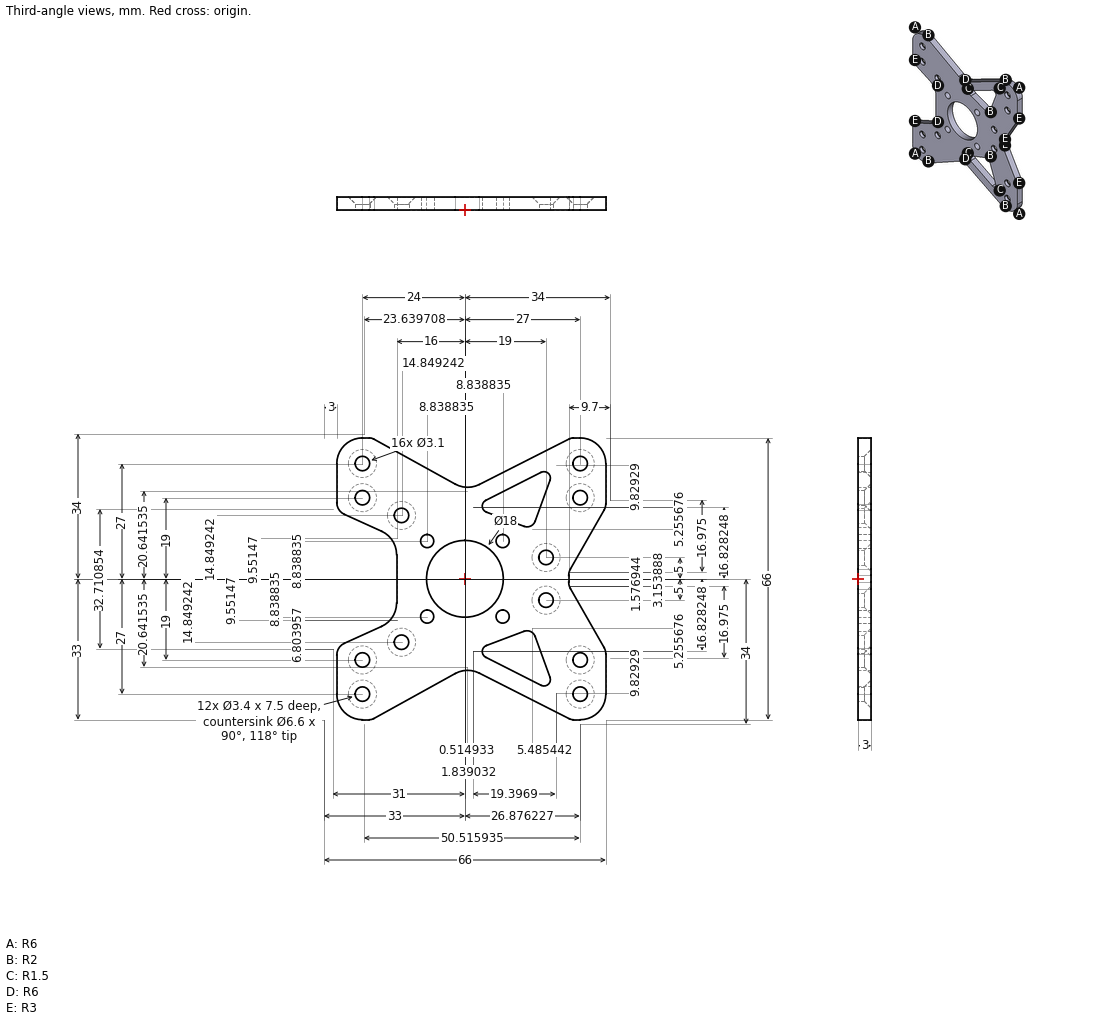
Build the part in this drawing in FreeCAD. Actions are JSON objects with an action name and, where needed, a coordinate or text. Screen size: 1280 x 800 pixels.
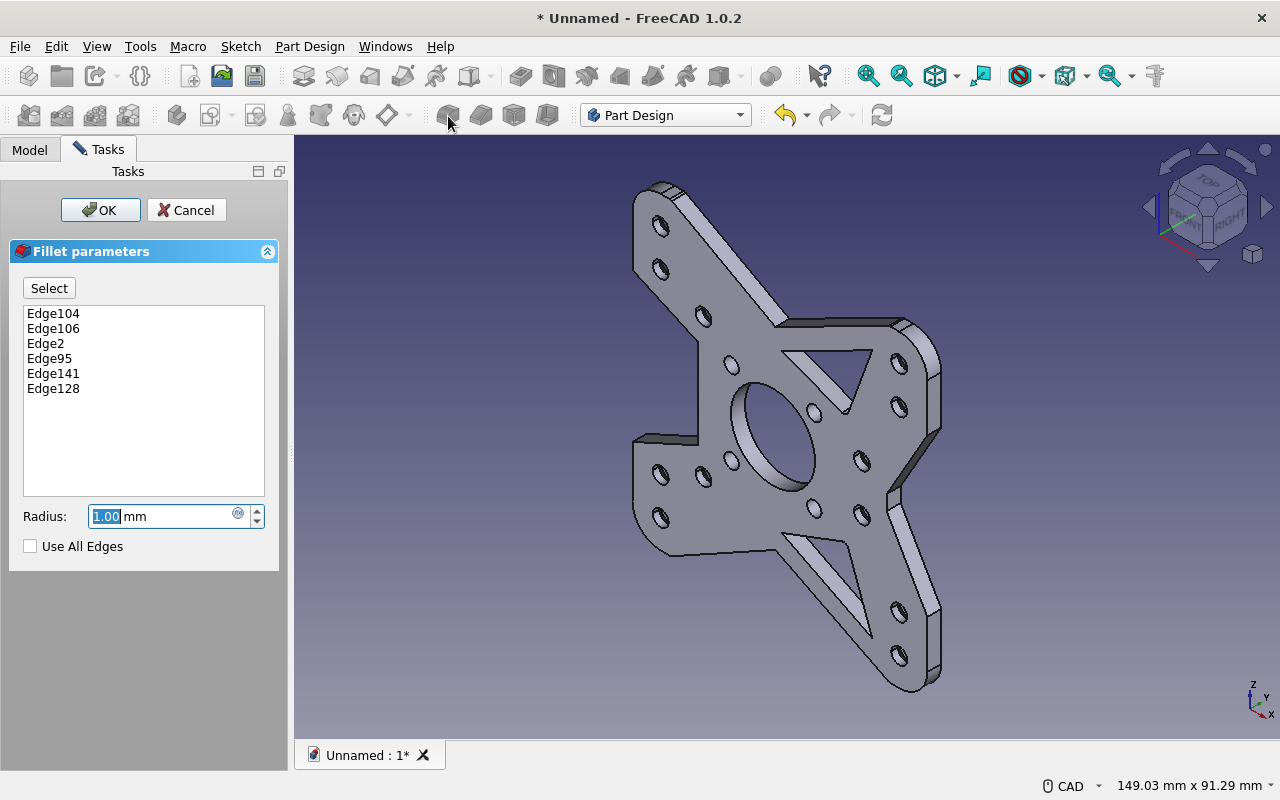
{"action": "type", "text": "2"}
{"action": "key", "text": "Tab"}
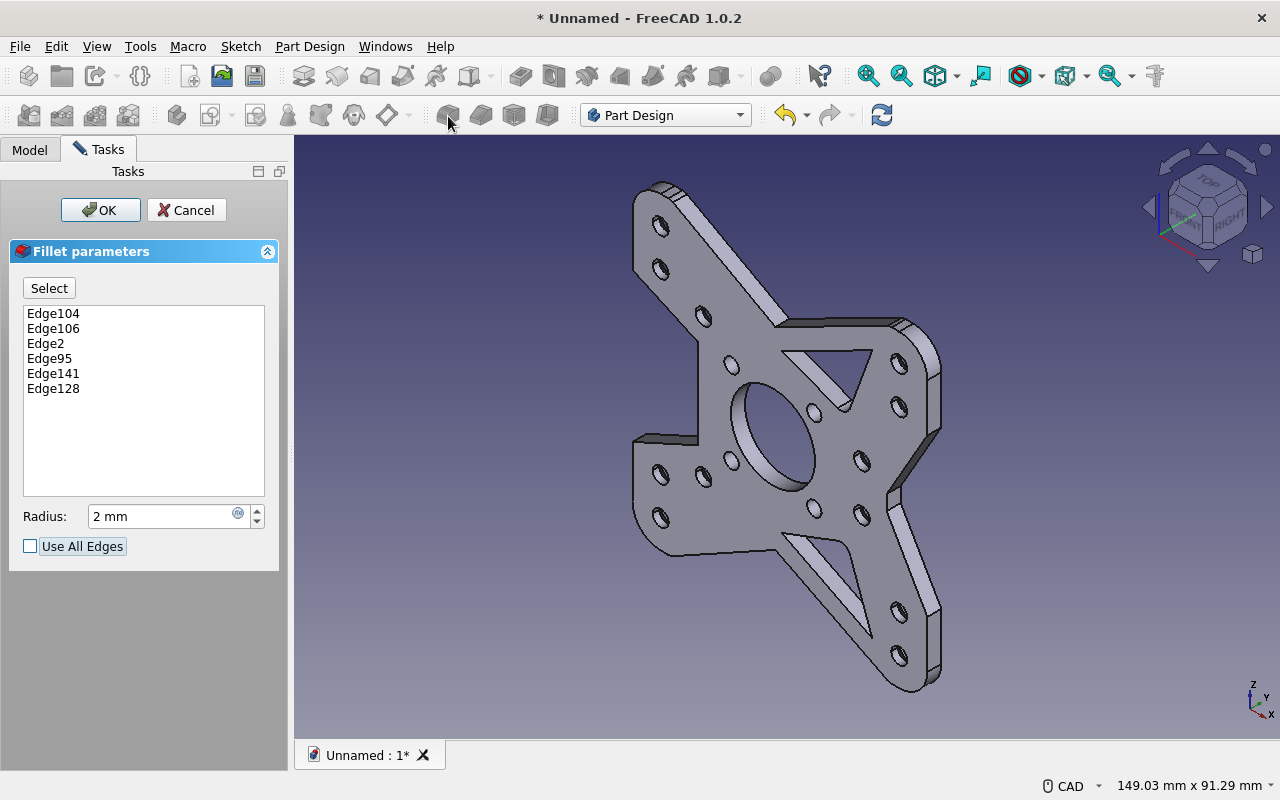
{"action": "left_click", "coordinate": [101, 210]}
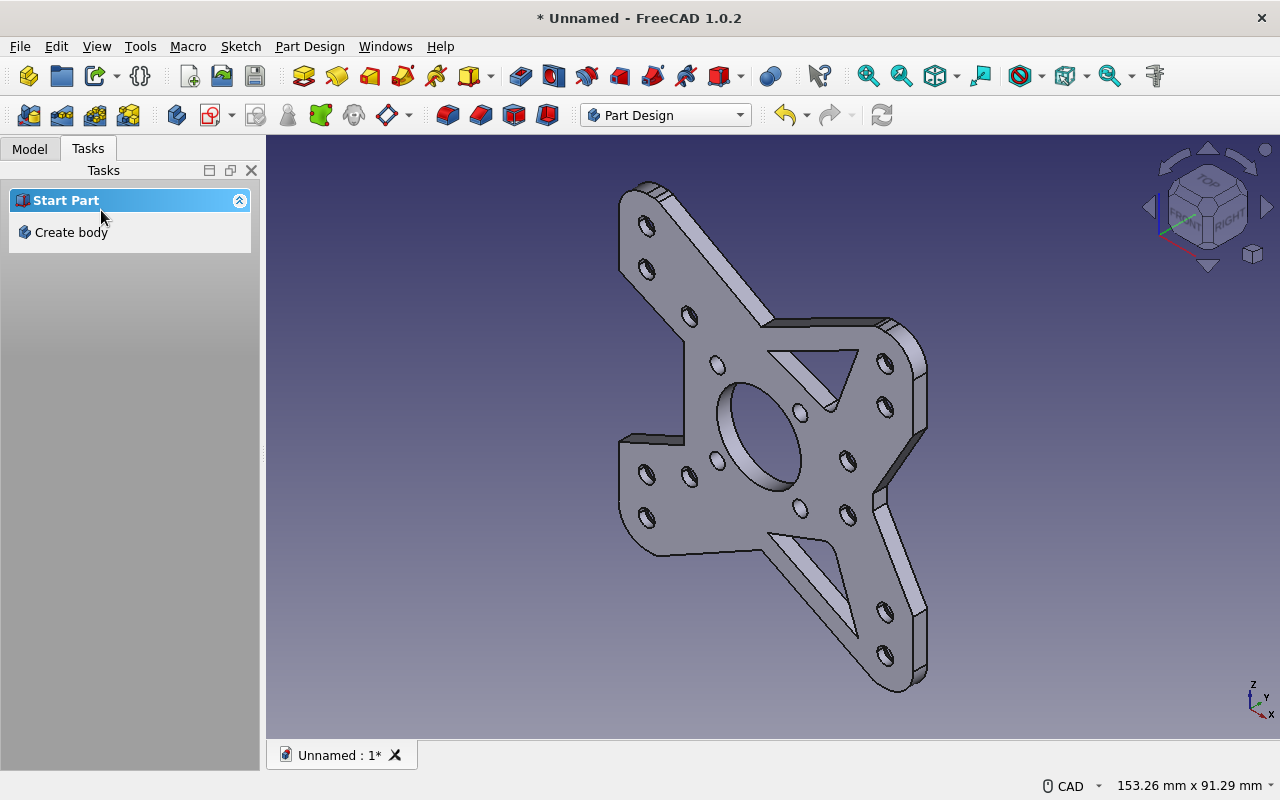
{"action": "scroll", "coordinate": [865, 345], "scroll_direction": "up", "scroll_amount": 4}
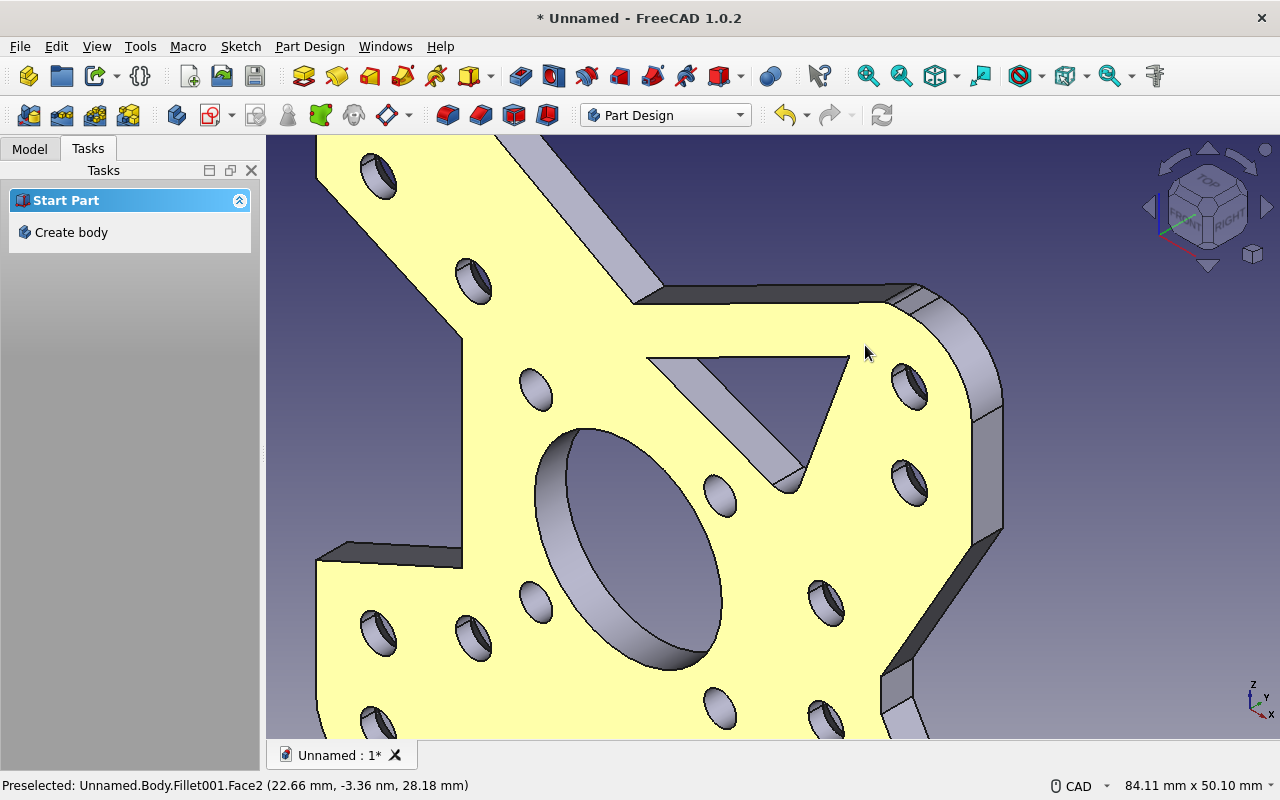
{"action": "key", "text": "v f"}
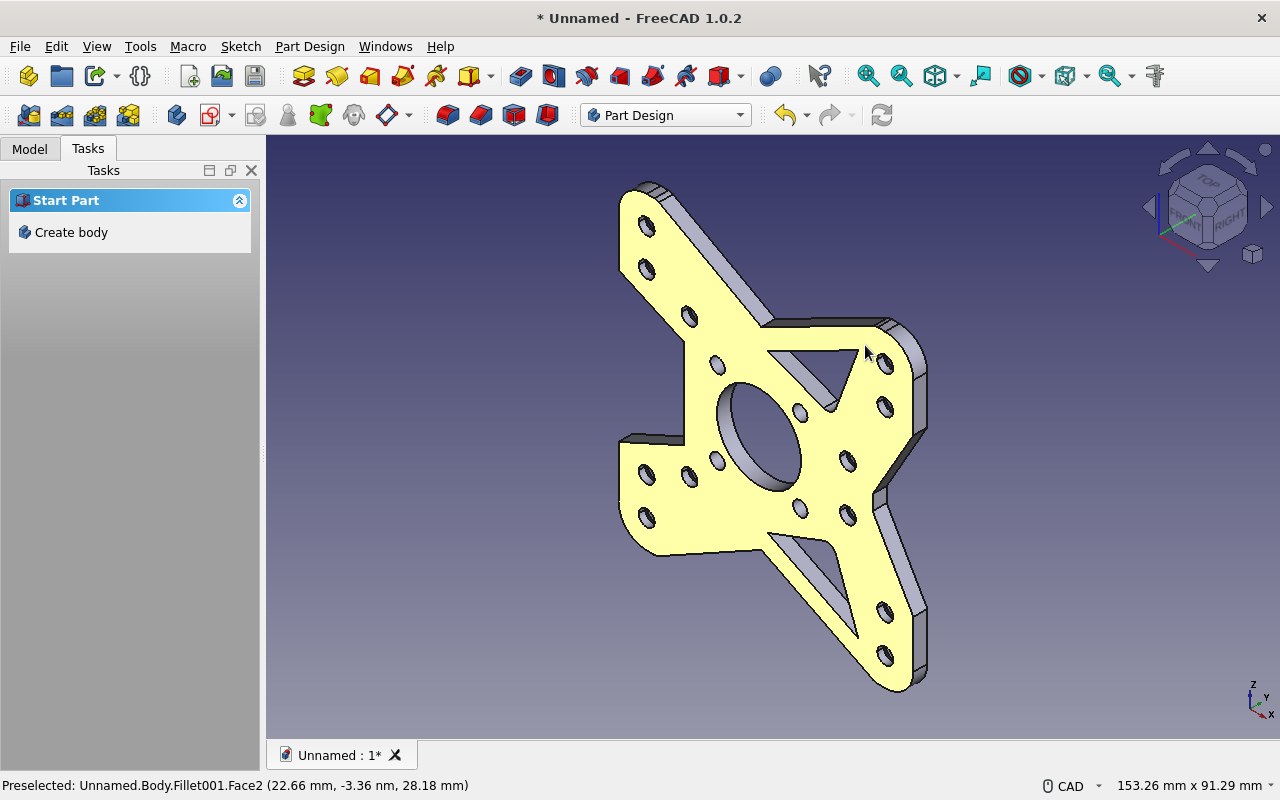
{"action": "key", "text": "2"}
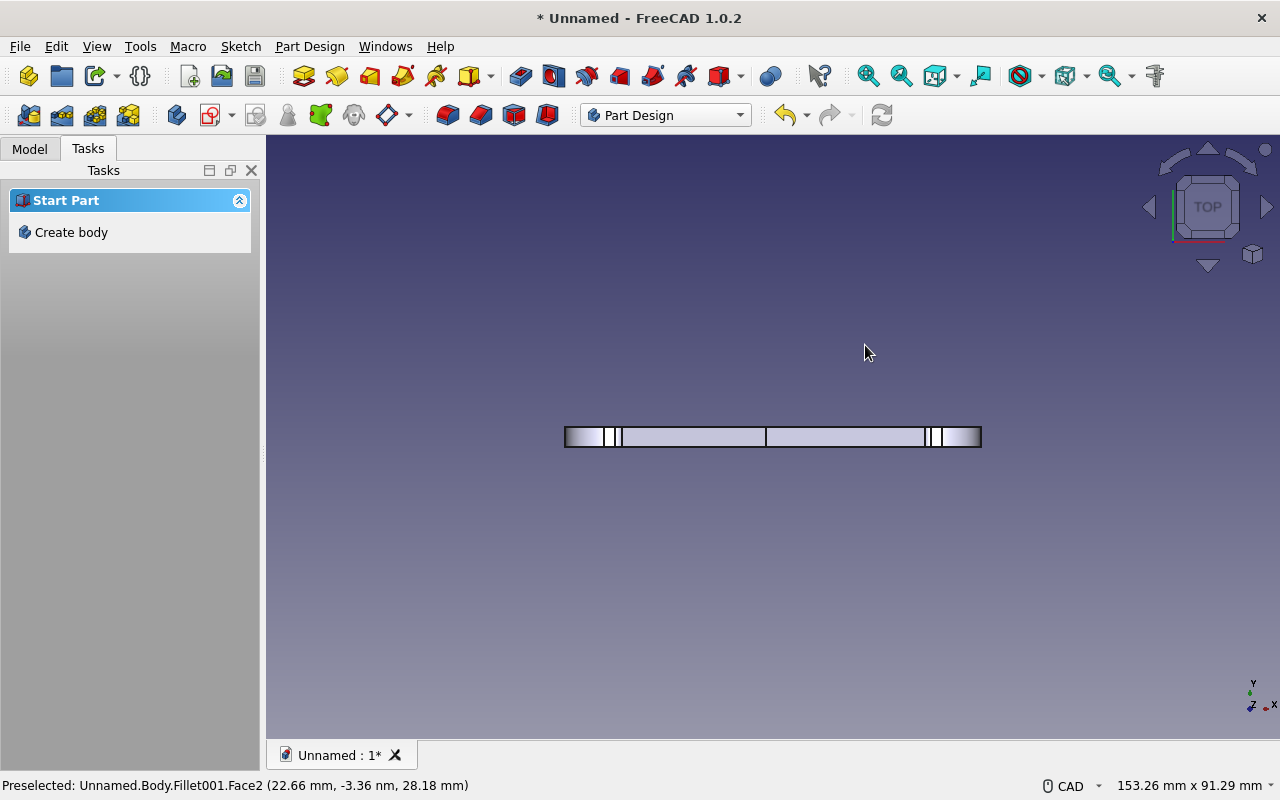
{"action": "key", "text": "v f"}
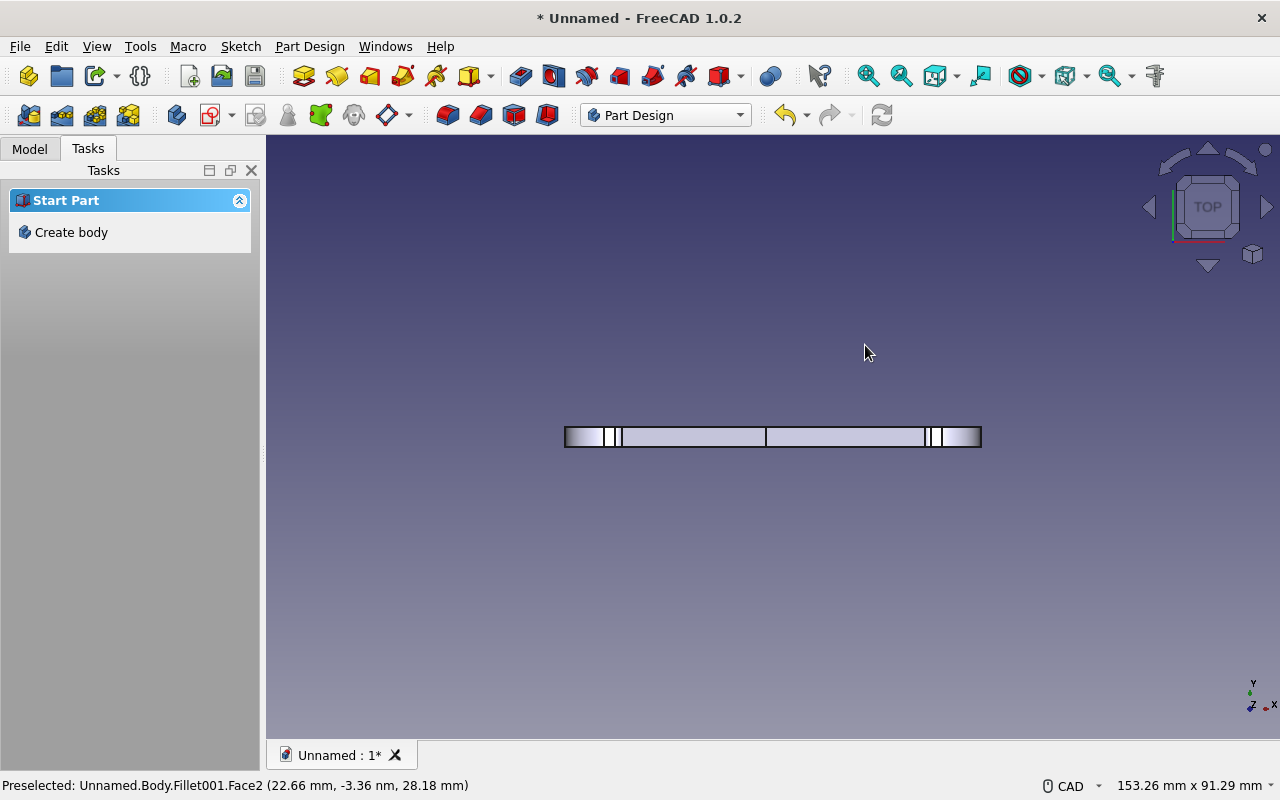
{"action": "scroll", "coordinate": [904, 436], "scroll_direction": "up", "scroll_amount": 4}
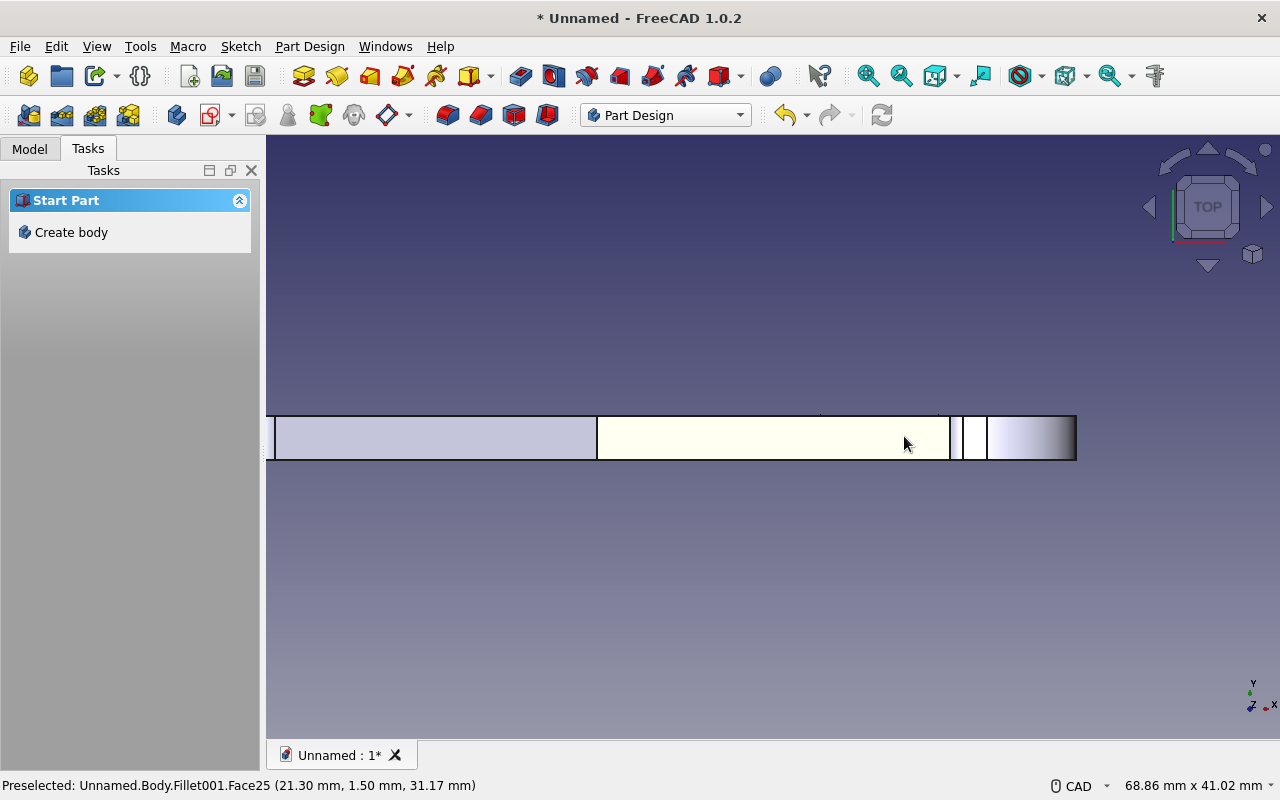
{"action": "left_click", "coordinate": [869, 76]}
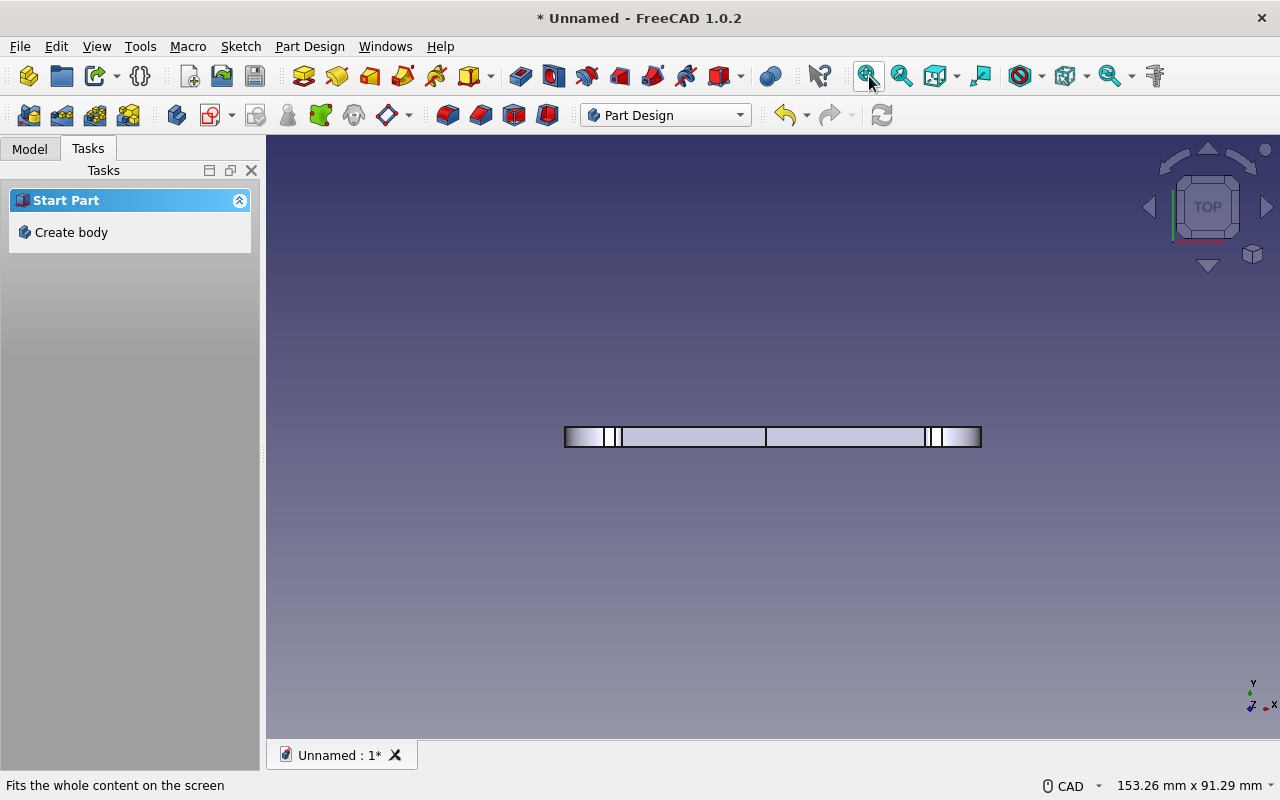
{"action": "key", "text": "0"}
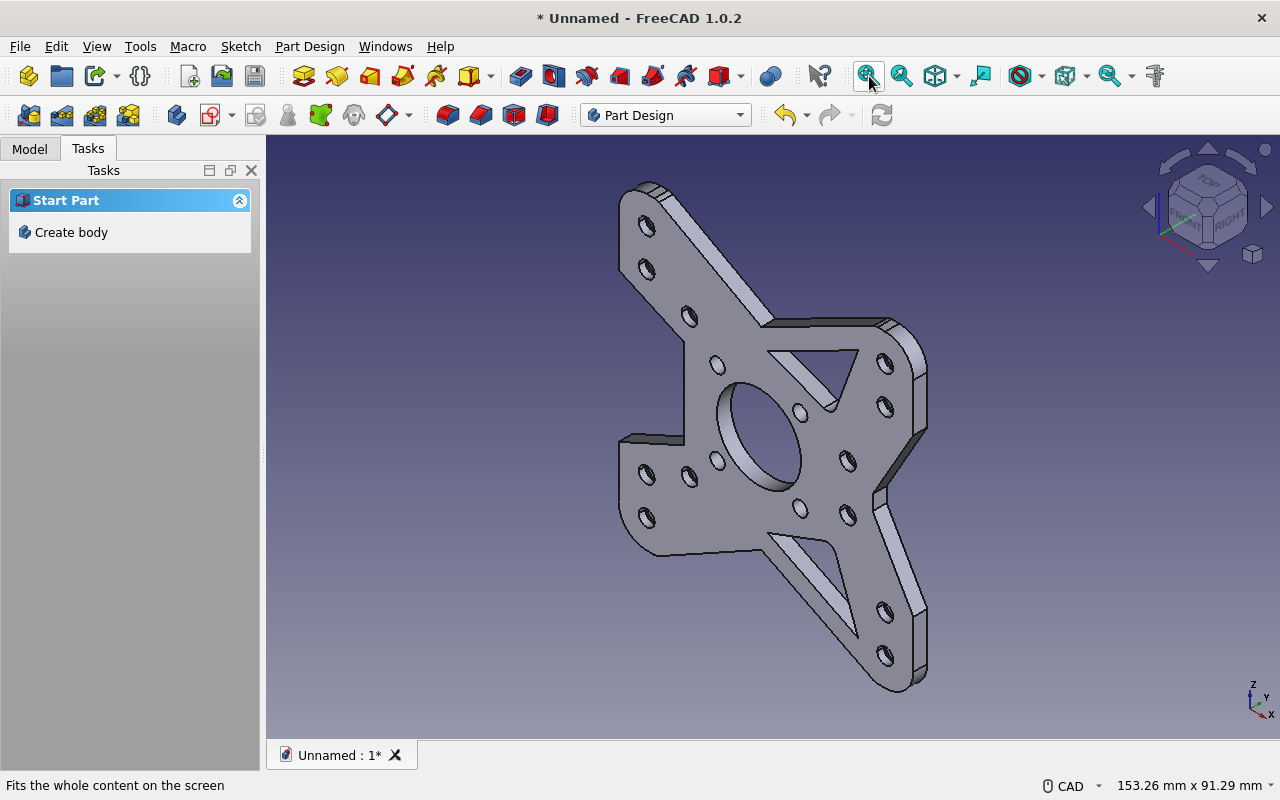
{"action": "scroll", "coordinate": [865, 345], "scroll_direction": "up", "scroll_amount": 4}